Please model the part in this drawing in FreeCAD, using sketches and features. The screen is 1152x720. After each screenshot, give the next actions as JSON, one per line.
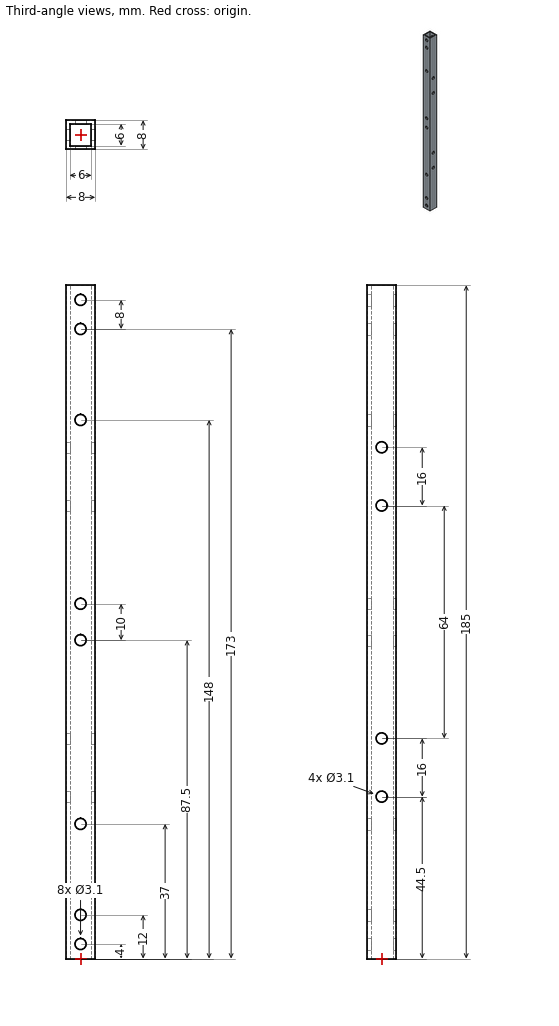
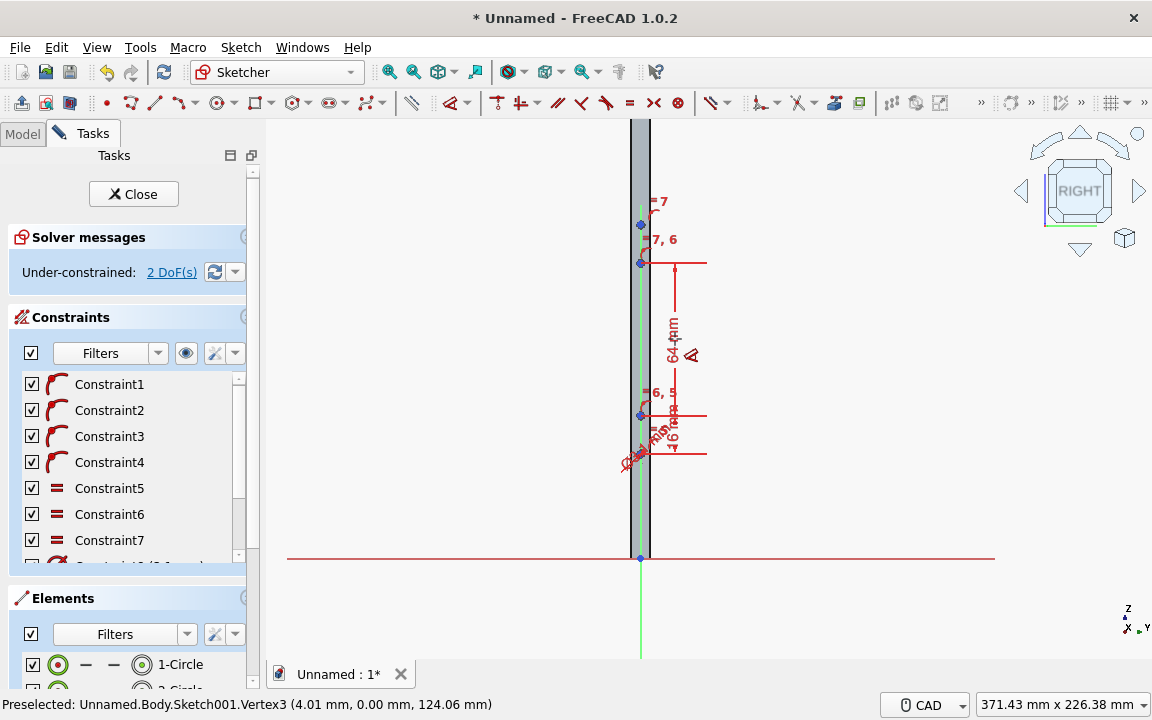
{"action": "left_click", "coordinate": [641, 263]}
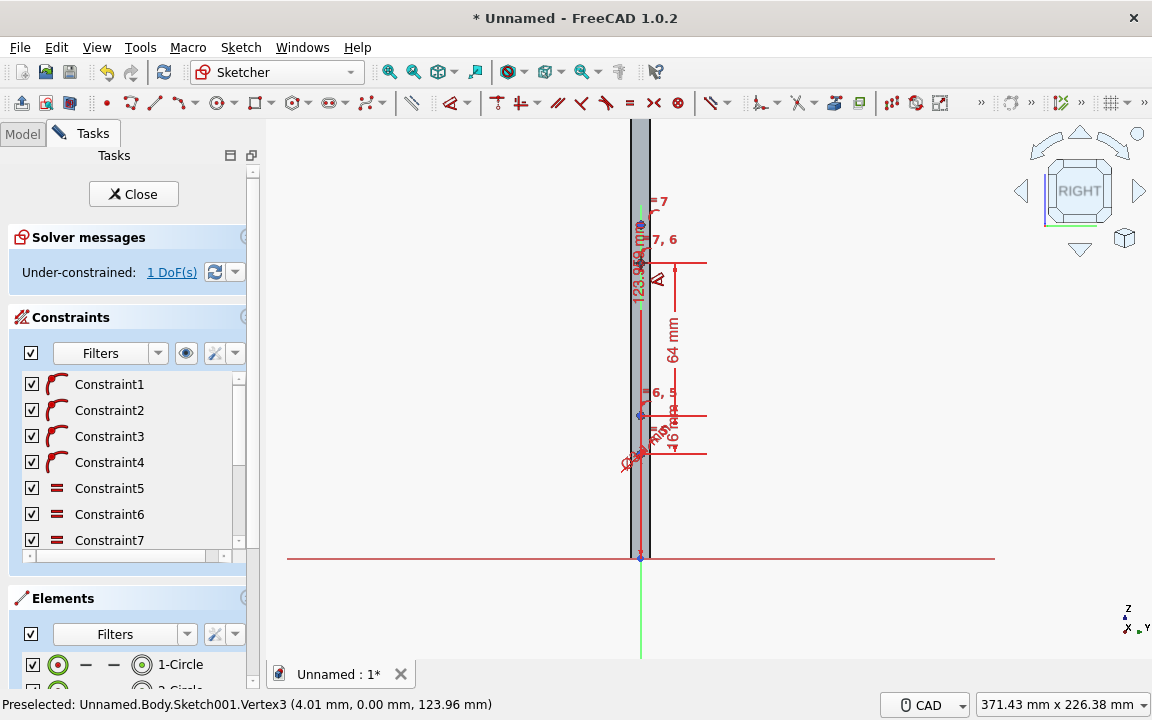
{"action": "left_click", "coordinate": [641, 225]}
{"action": "left_click", "coordinate": [675, 244]}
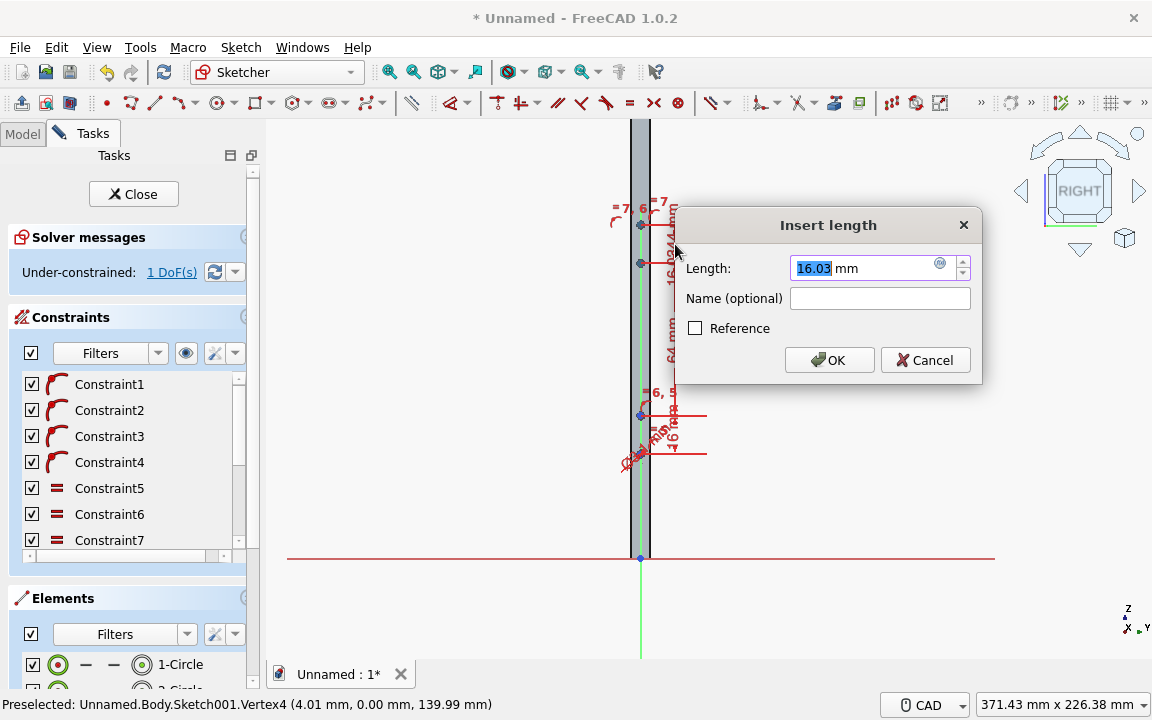
{"action": "type", "text": "16"}
{"action": "key", "text": "Return"}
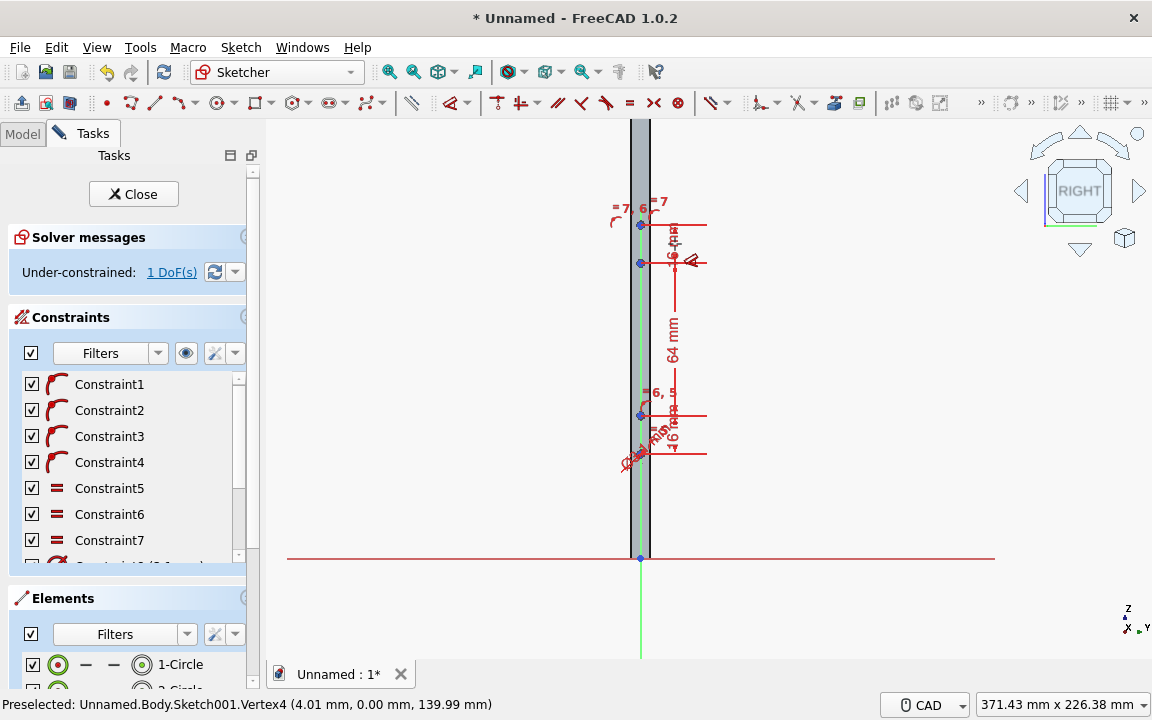
{"action": "left_click", "coordinate": [641, 454]}
{"action": "left_click", "coordinate": [675, 507]}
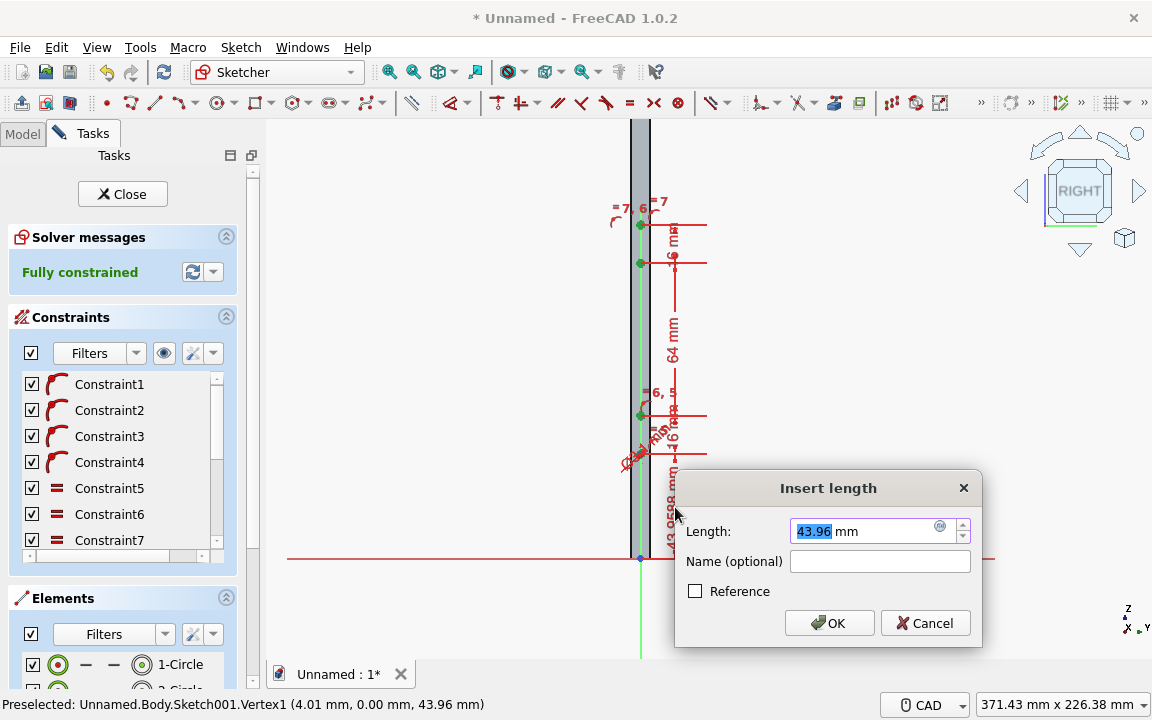
{"action": "type", "text": "44.5"}
{"action": "key", "text": "Return"}
{"action": "key", "text": "Escape"}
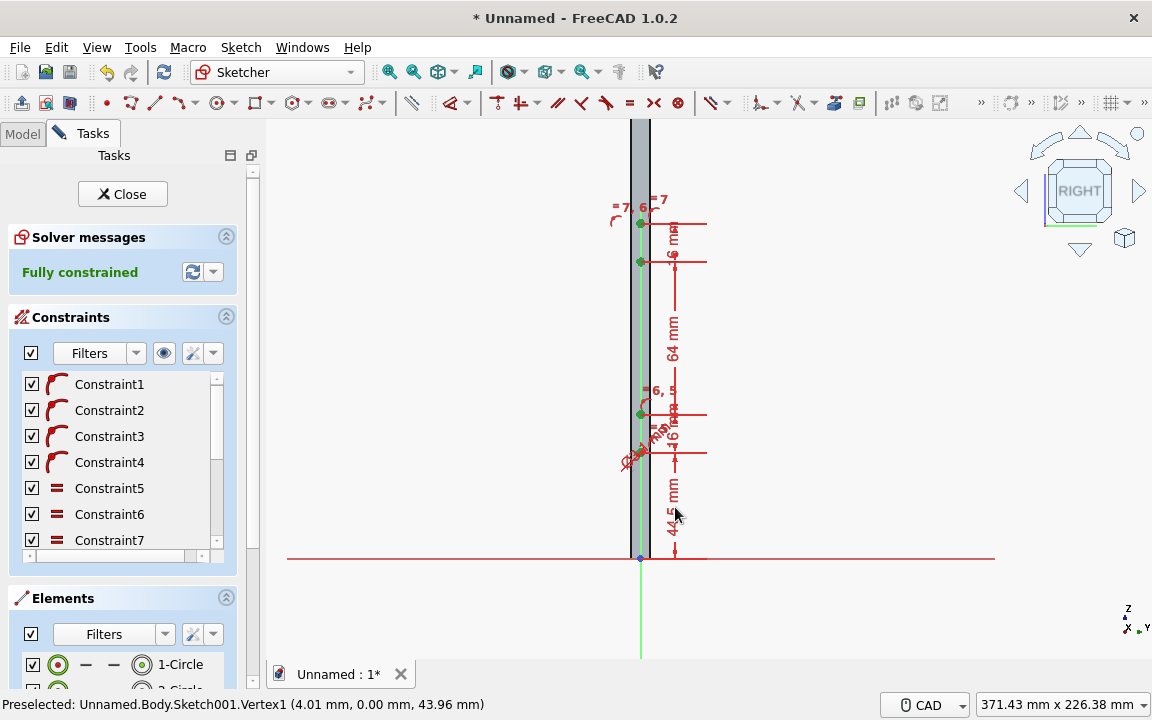
{"action": "left_click", "coordinate": [123, 194]}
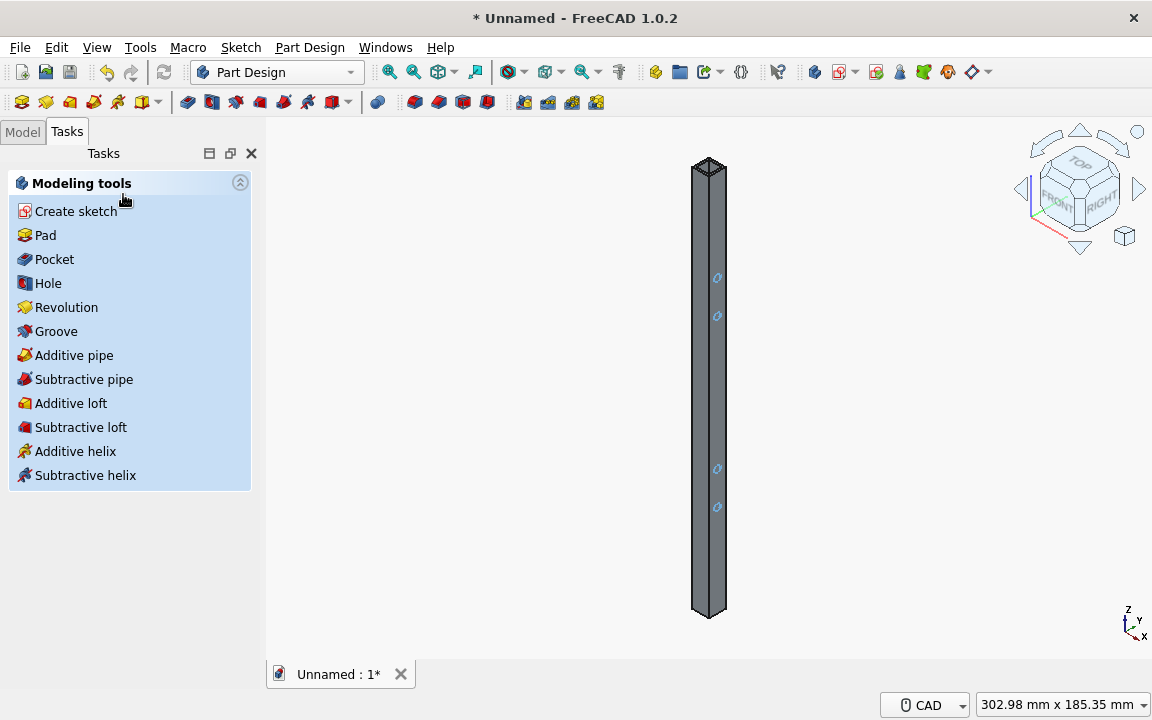
{"action": "left_click", "coordinate": [188, 102]}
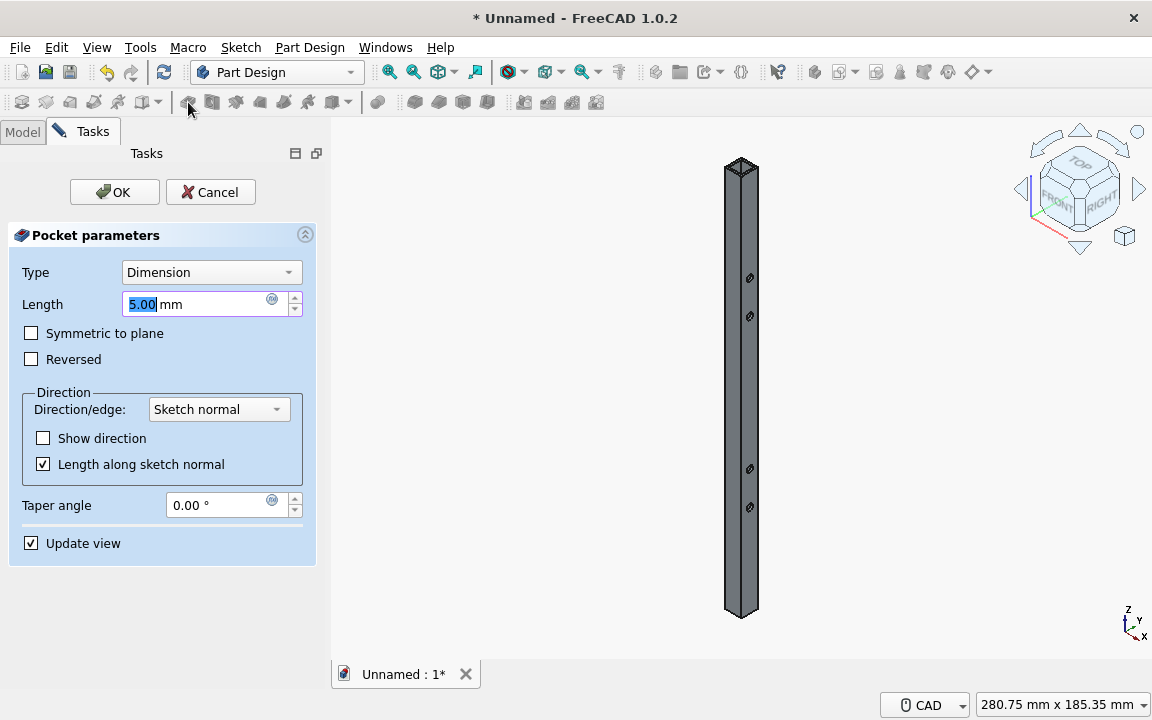
{"action": "left_click", "coordinate": [212, 272]}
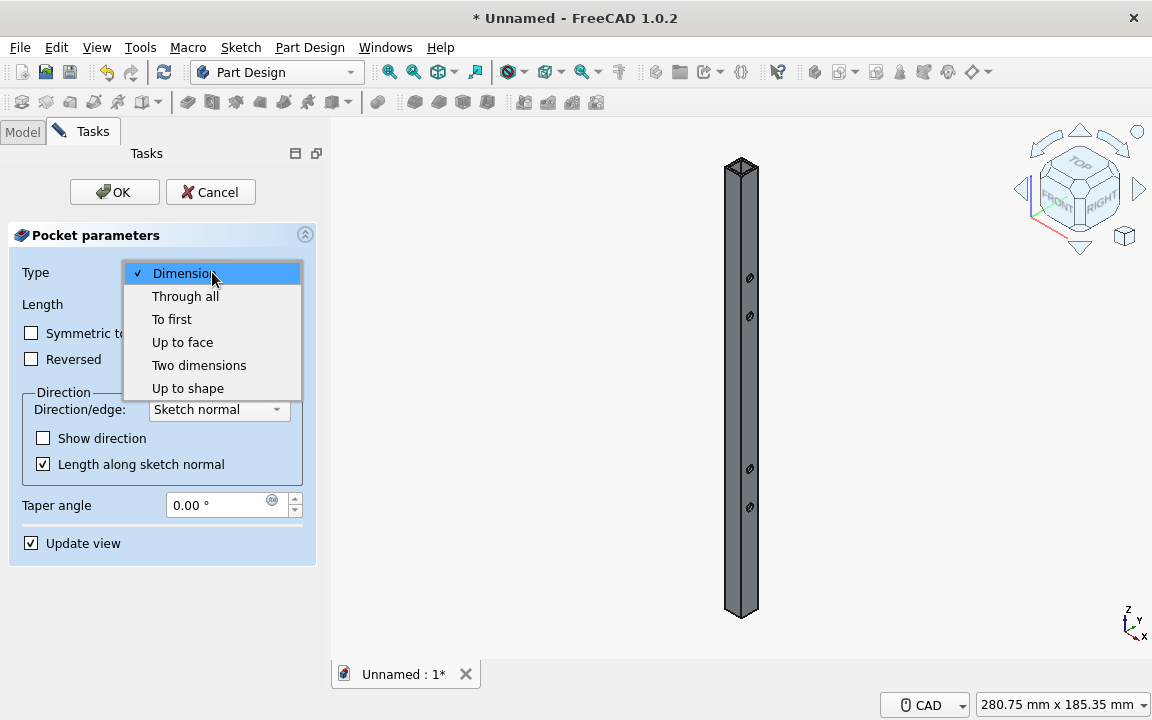
{"action": "left_click", "coordinate": [212, 296]}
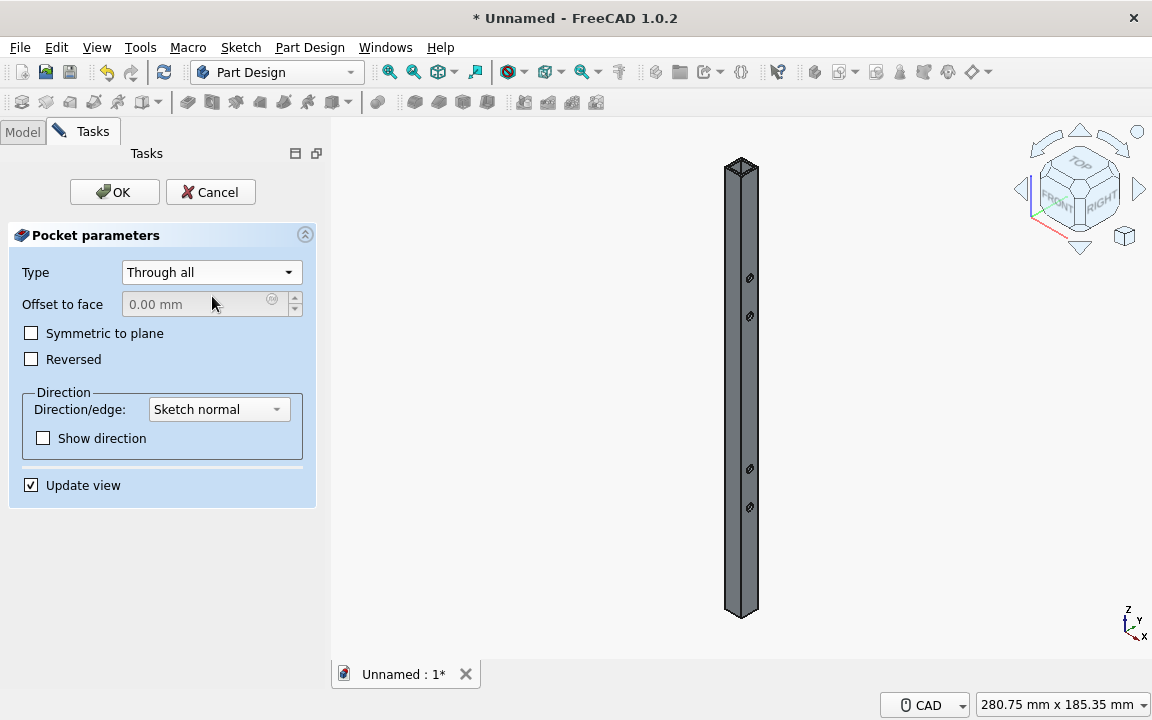
{"action": "left_click", "coordinate": [115, 192]}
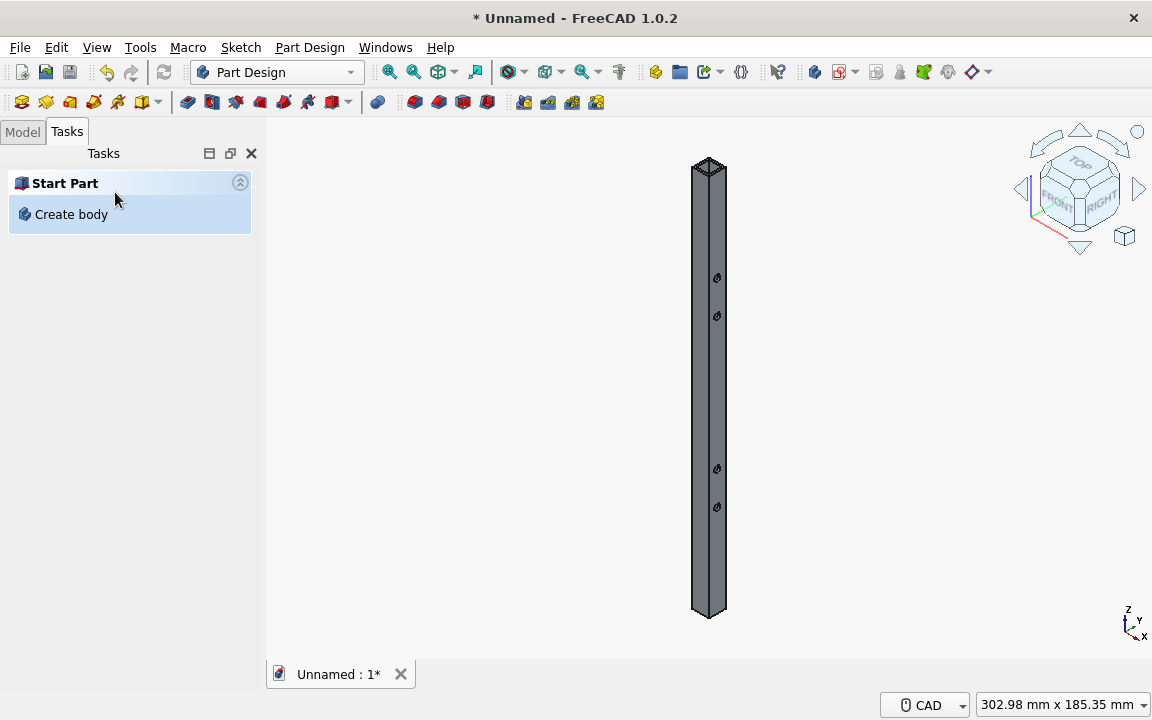
{"action": "key", "text": "4"}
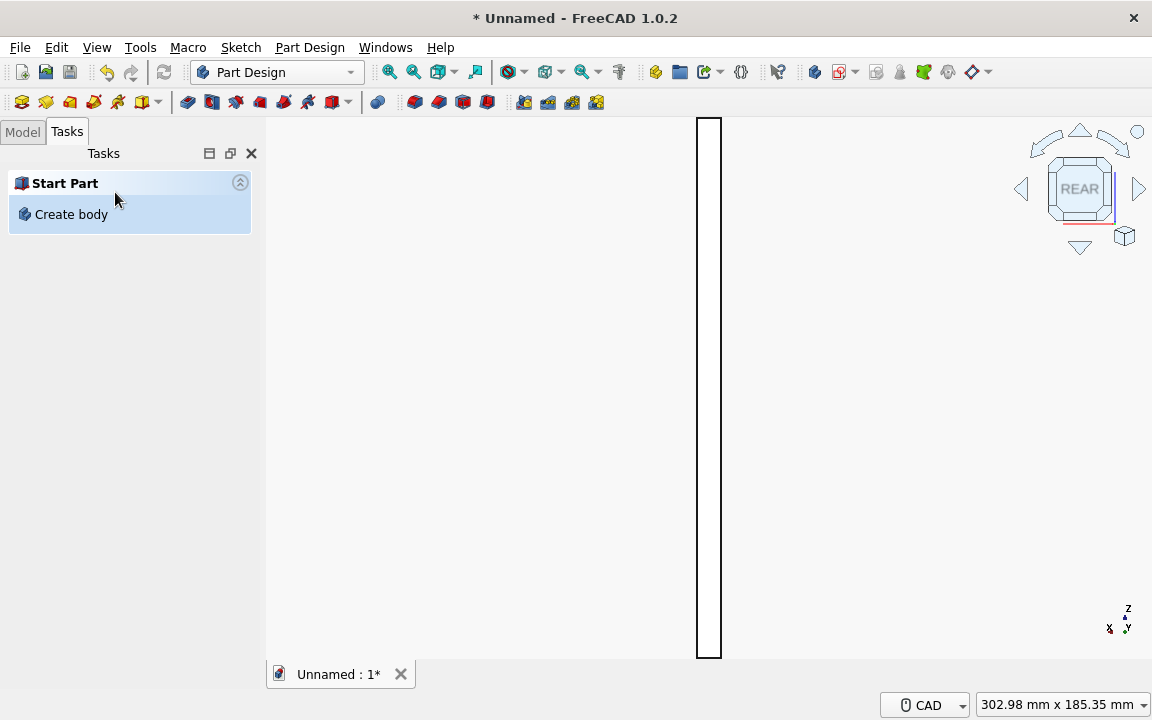
{"action": "left_click", "coordinate": [709, 155]}